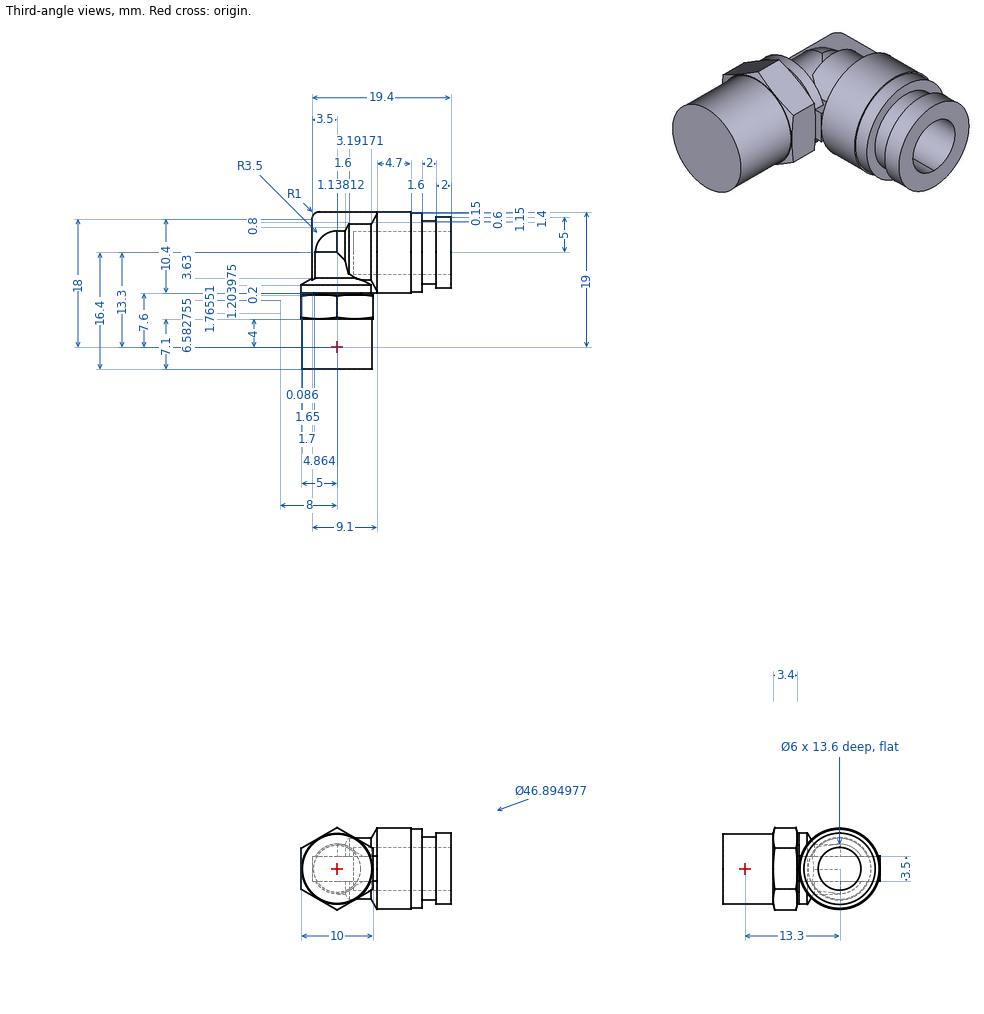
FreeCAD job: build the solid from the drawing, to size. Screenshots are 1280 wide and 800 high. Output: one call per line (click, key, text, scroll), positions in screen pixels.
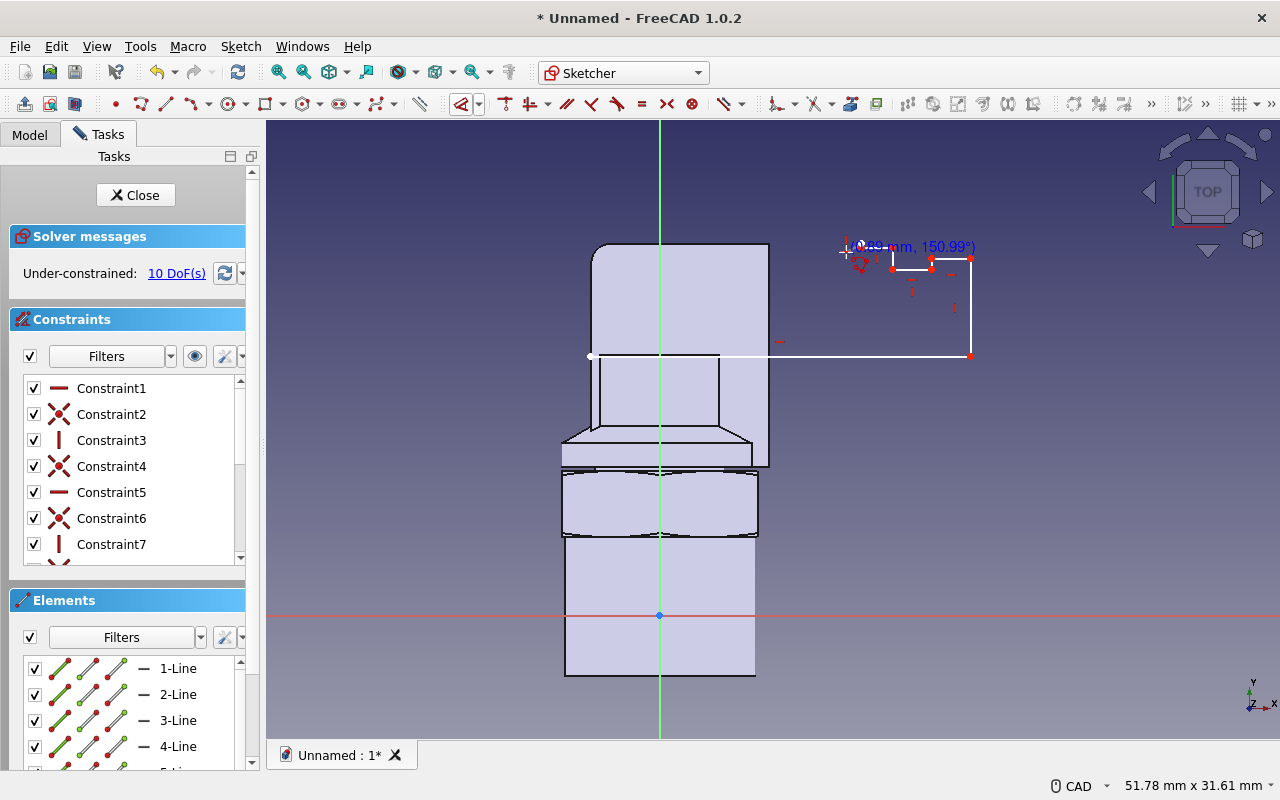
click(769, 244)
click(754, 271)
click(691, 271)
click(682, 287)
click(660, 287)
right_click(660, 287)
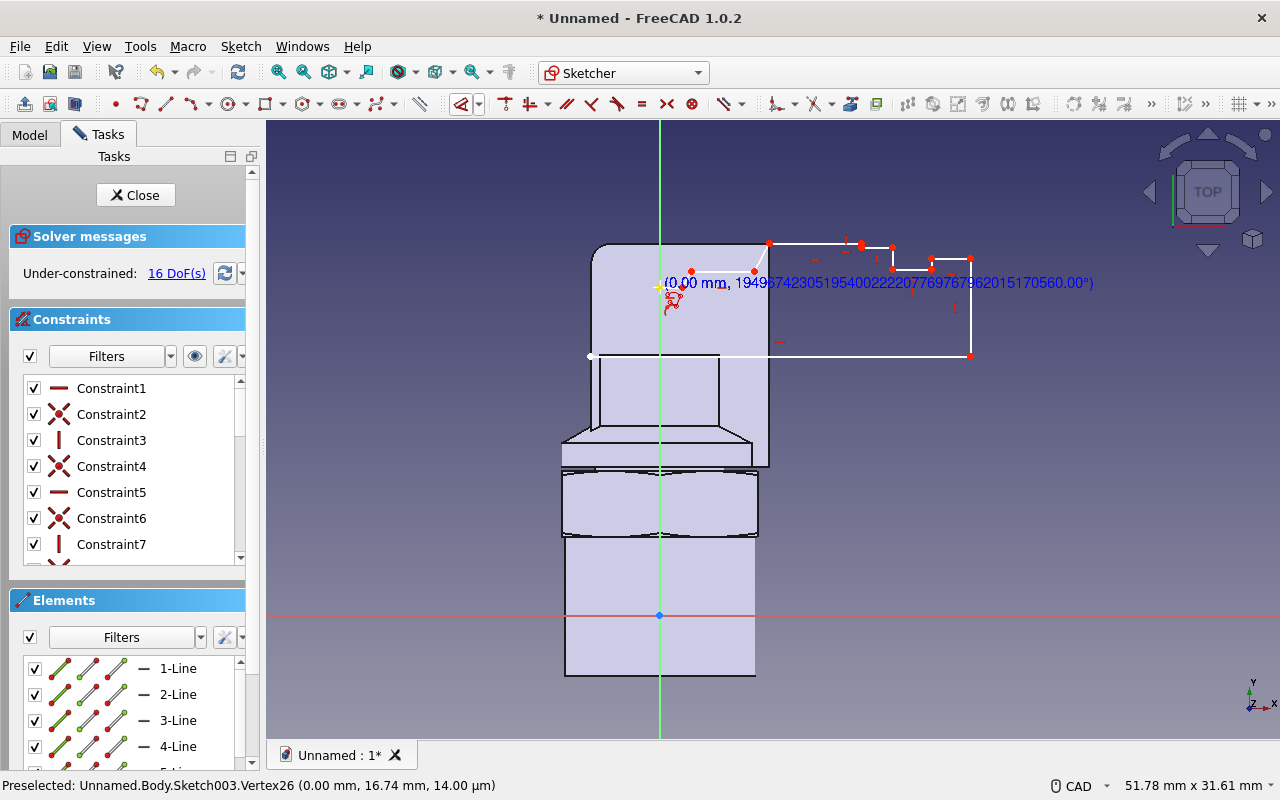
click(190, 104)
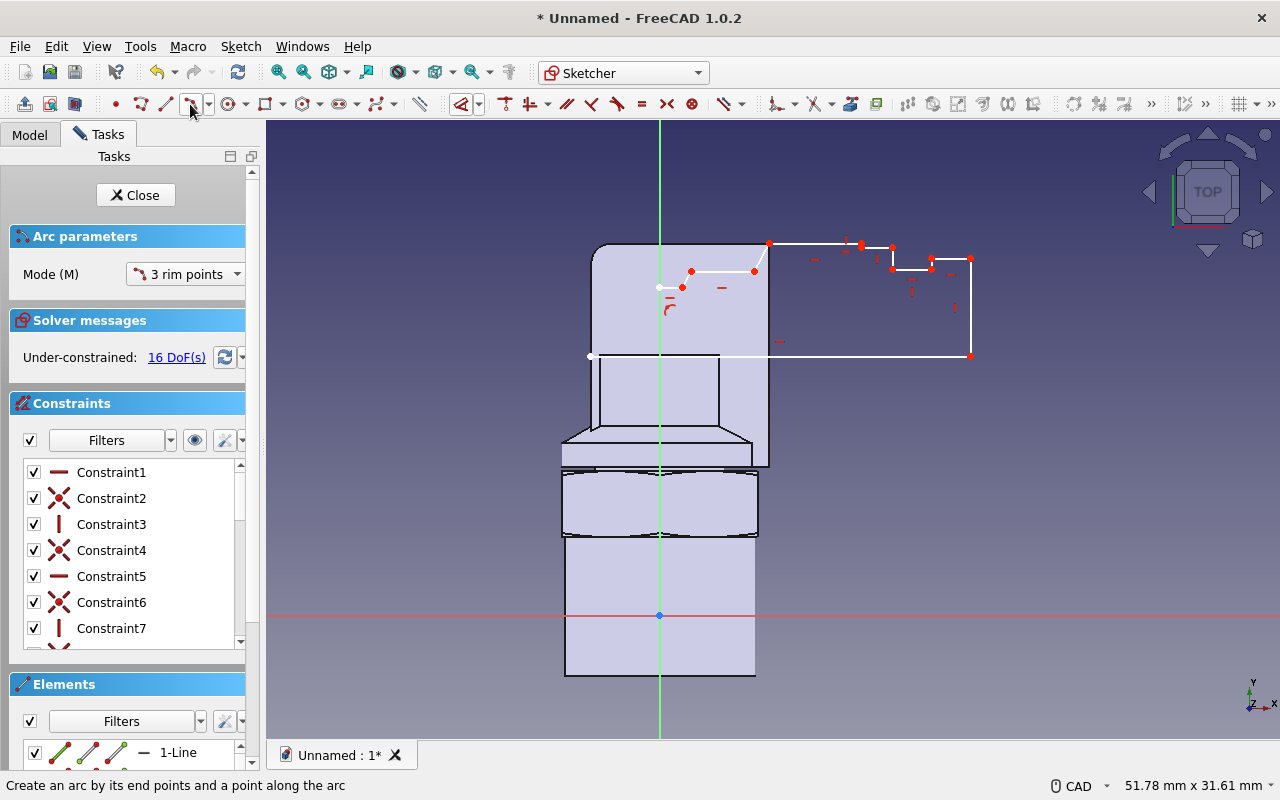
scroll(660, 287, up, 2)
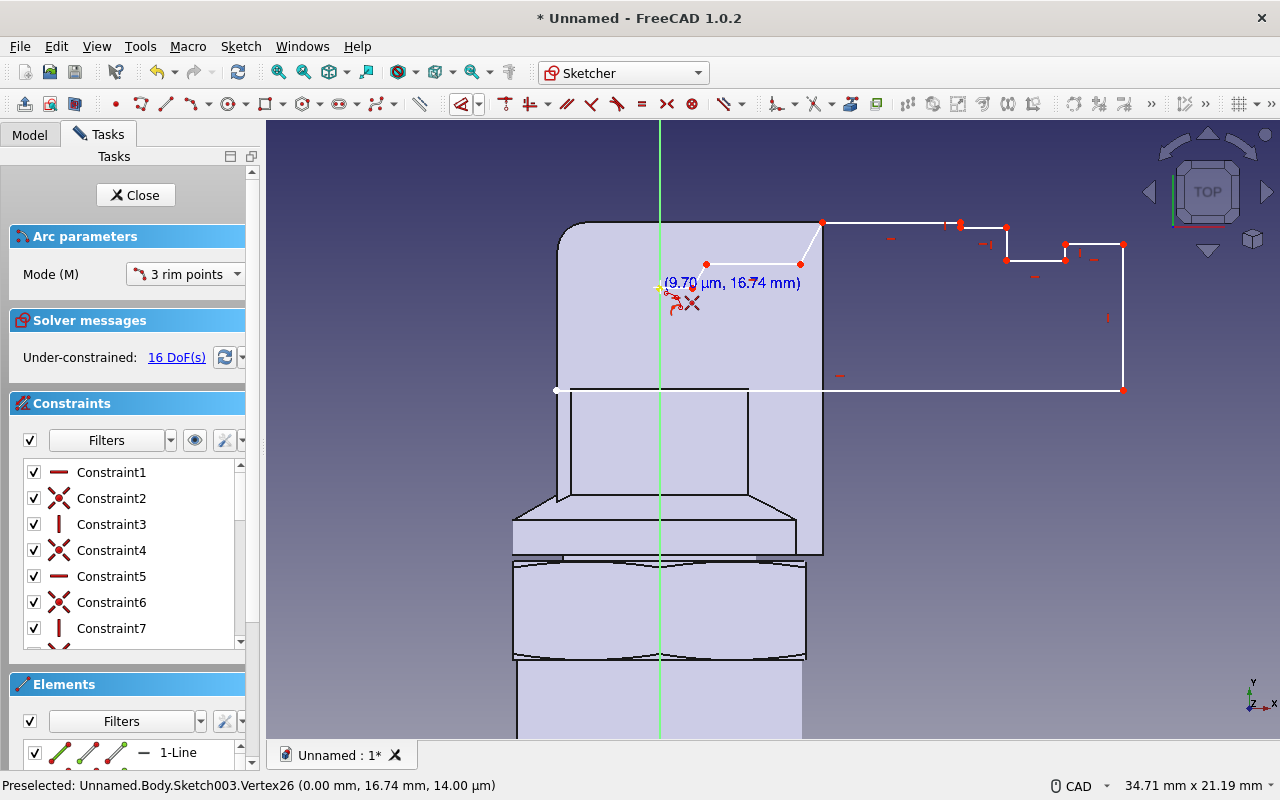
click(660, 288)
click(557, 391)
click(587, 317)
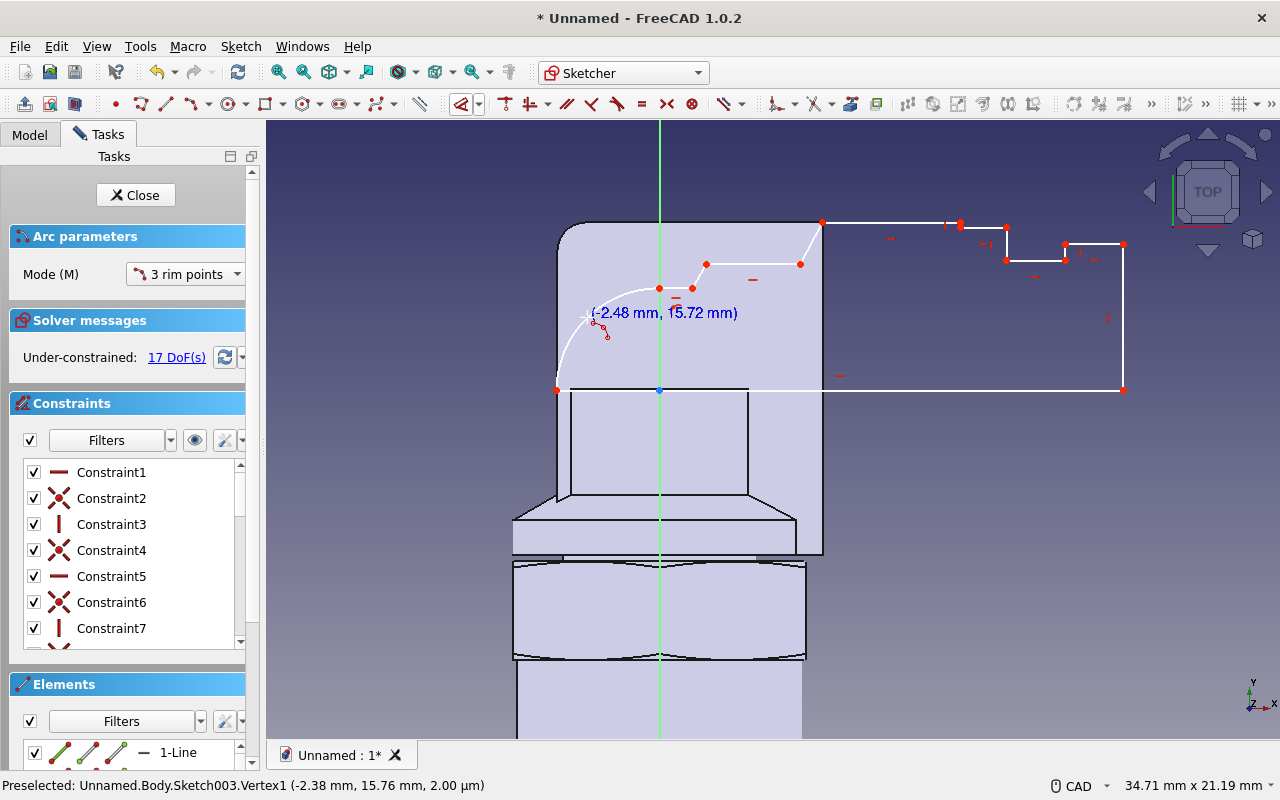
key(g)
key(l)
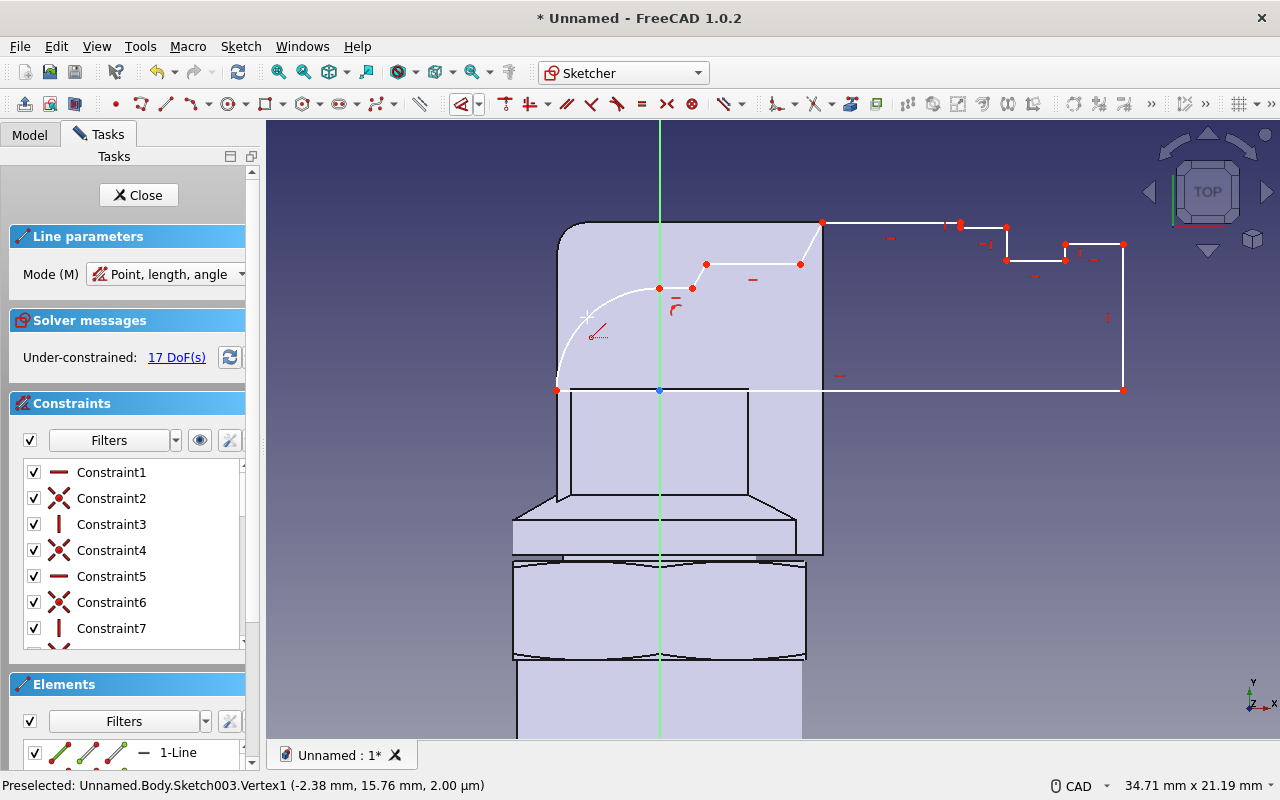
click(501, 389)
click(331, 389)
key(Escape)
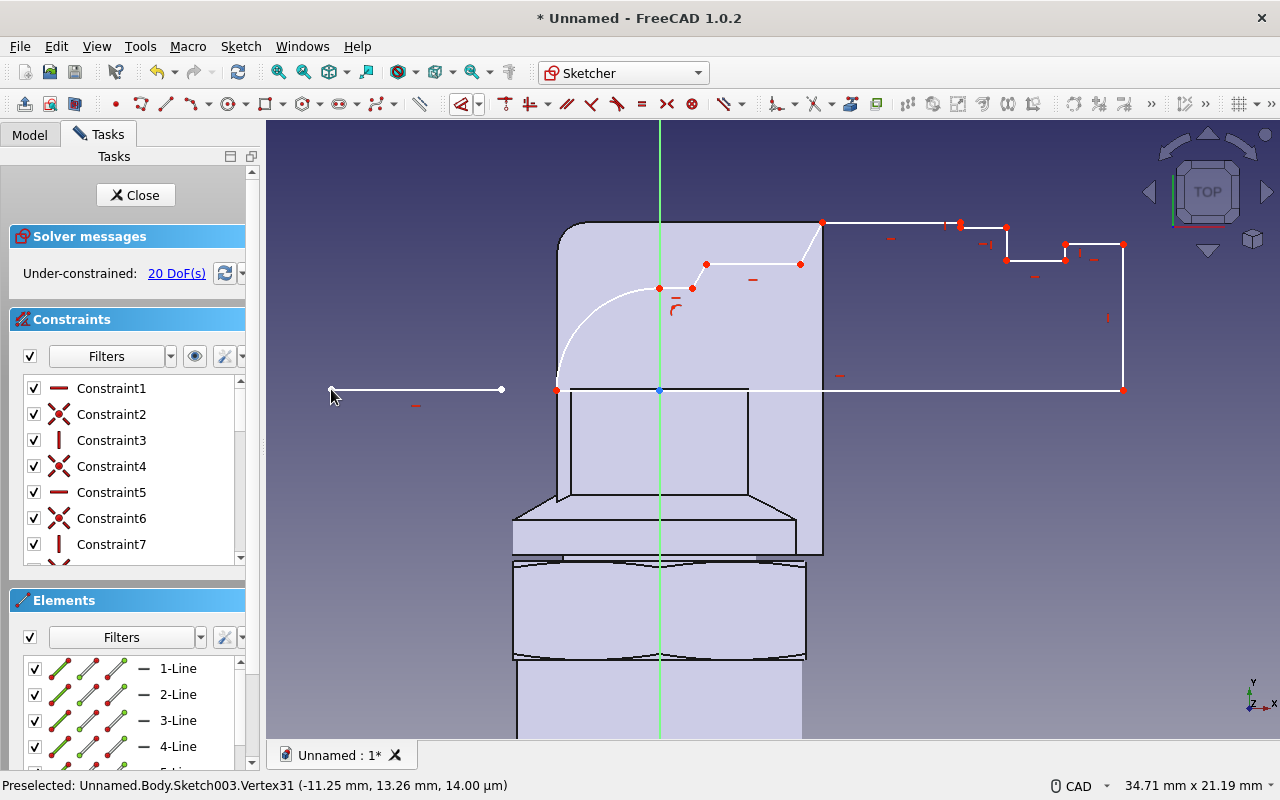
click(450, 390)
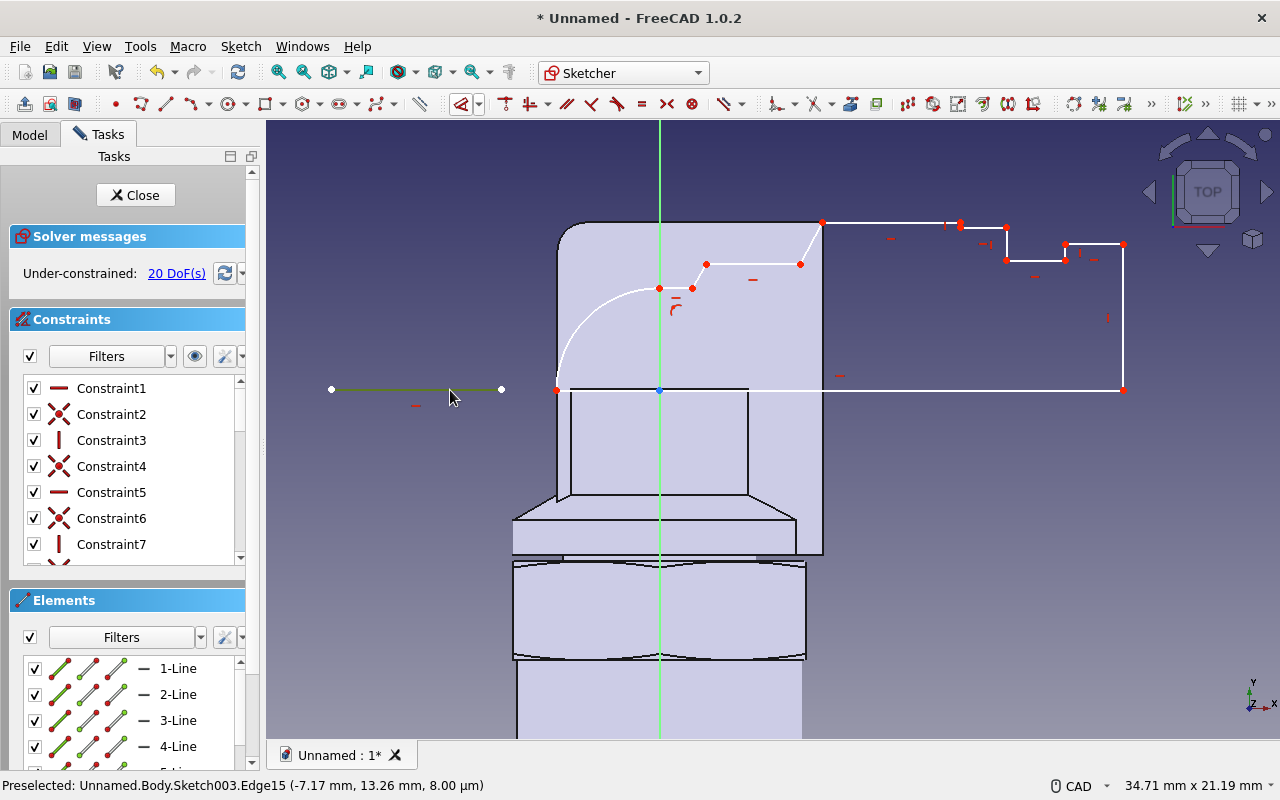
key(g)
key(n)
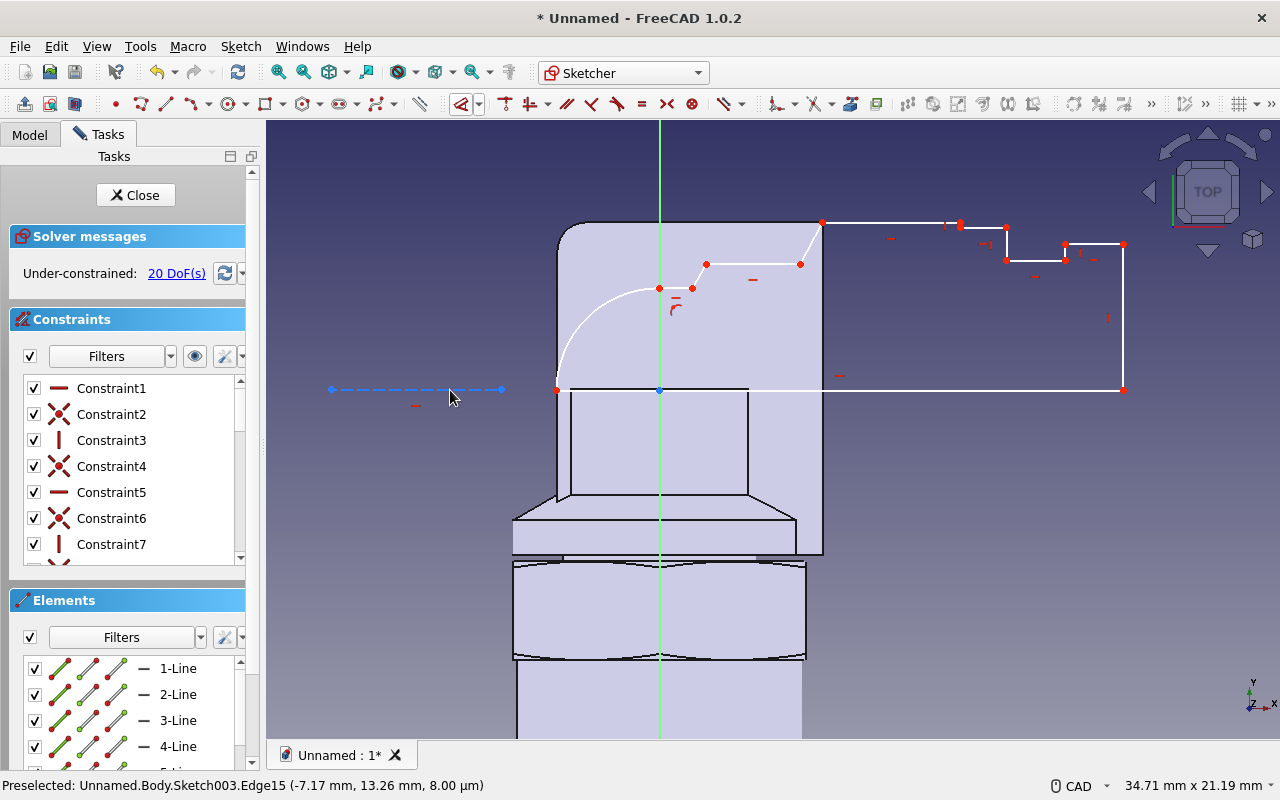
scroll(683, 288, up, 2)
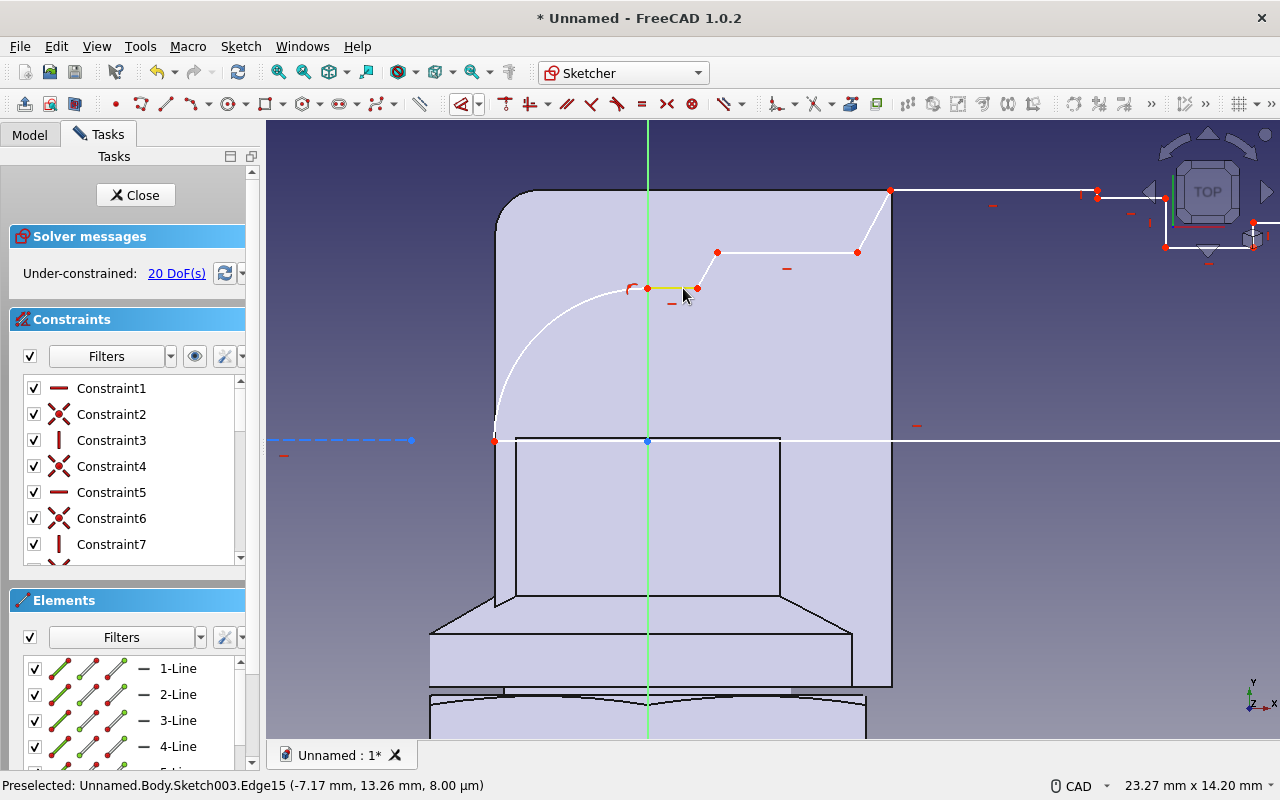
click(682, 288)